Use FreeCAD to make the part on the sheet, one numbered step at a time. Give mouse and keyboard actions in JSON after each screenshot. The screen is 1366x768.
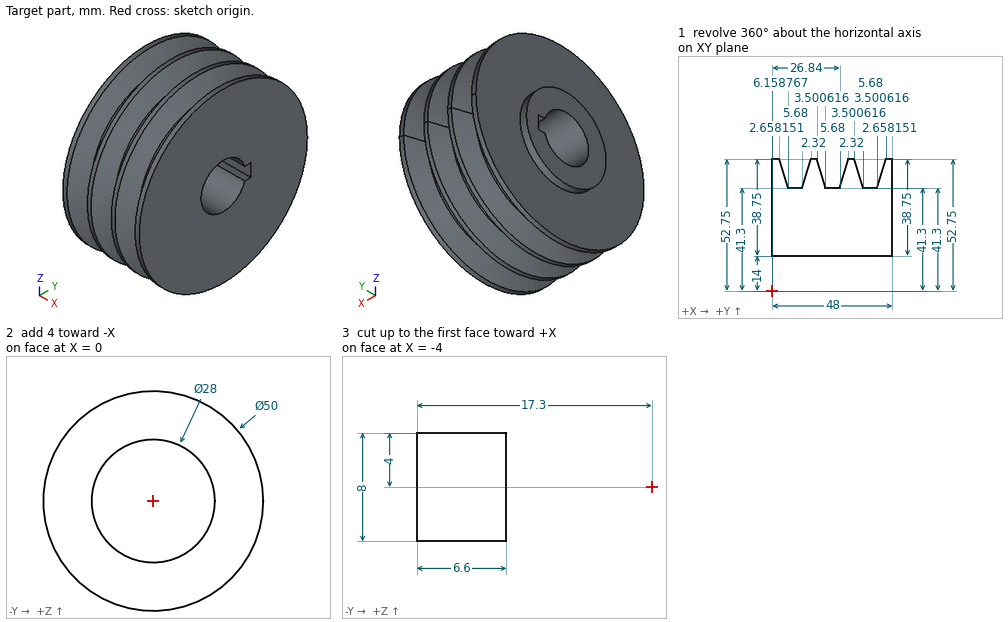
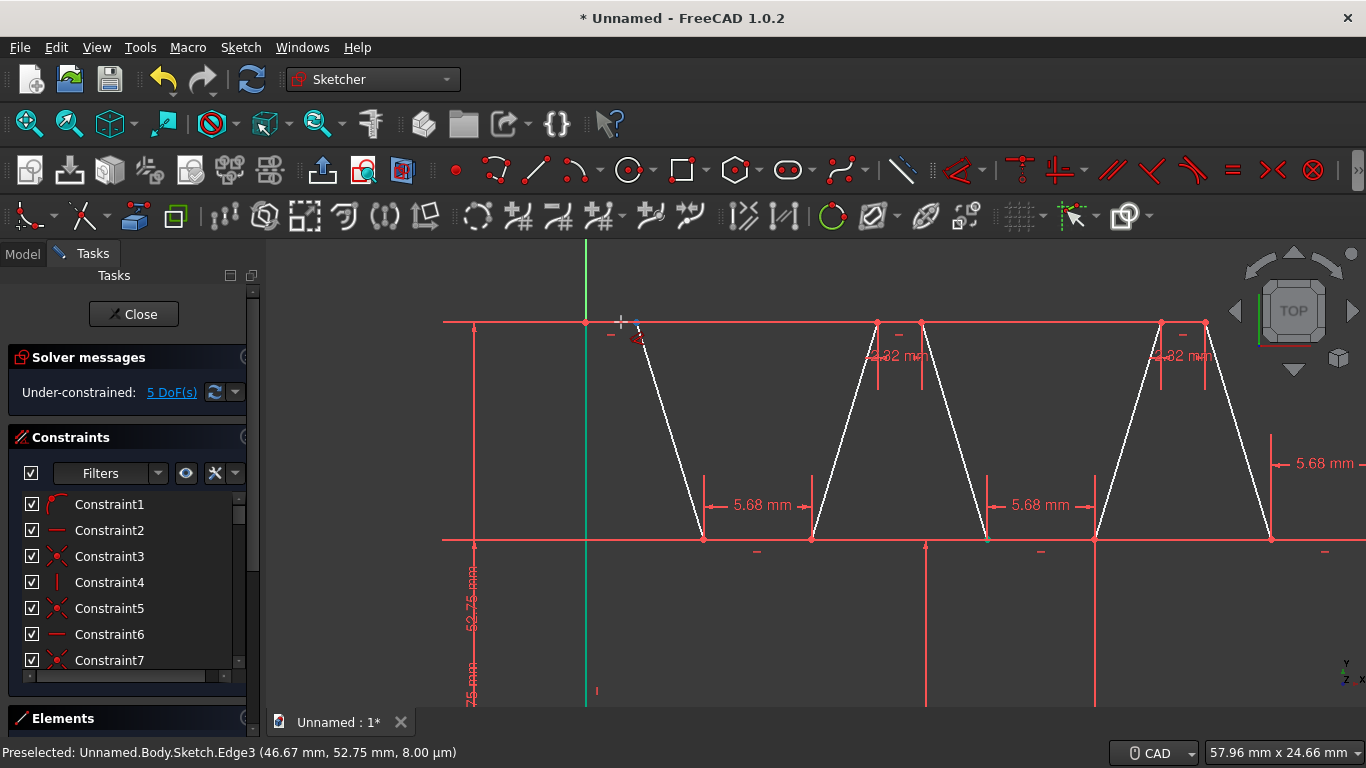
{"action": "left_click", "coordinate": [621, 322]}
{"action": "left_click", "coordinate": [611, 288]}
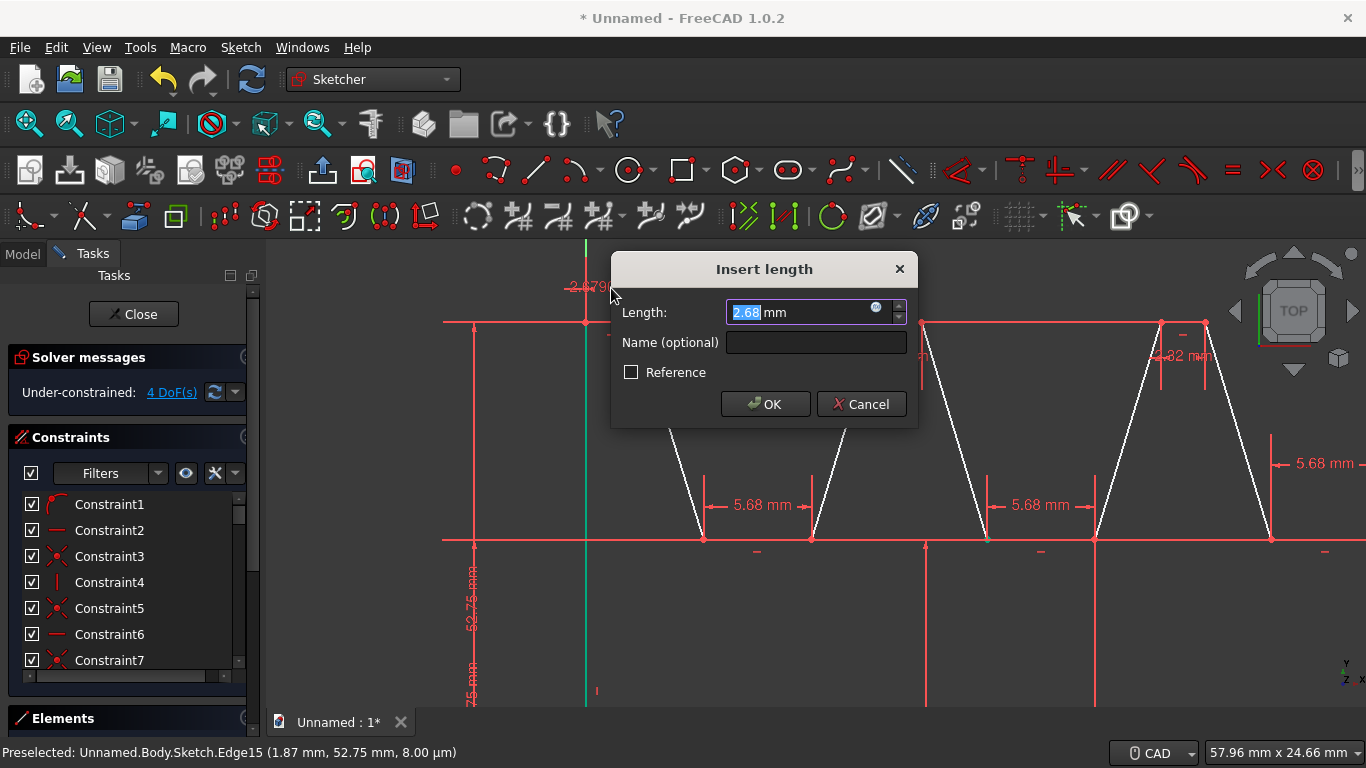
{"action": "type", "text": "2.658151"}
{"action": "key", "text": "Return"}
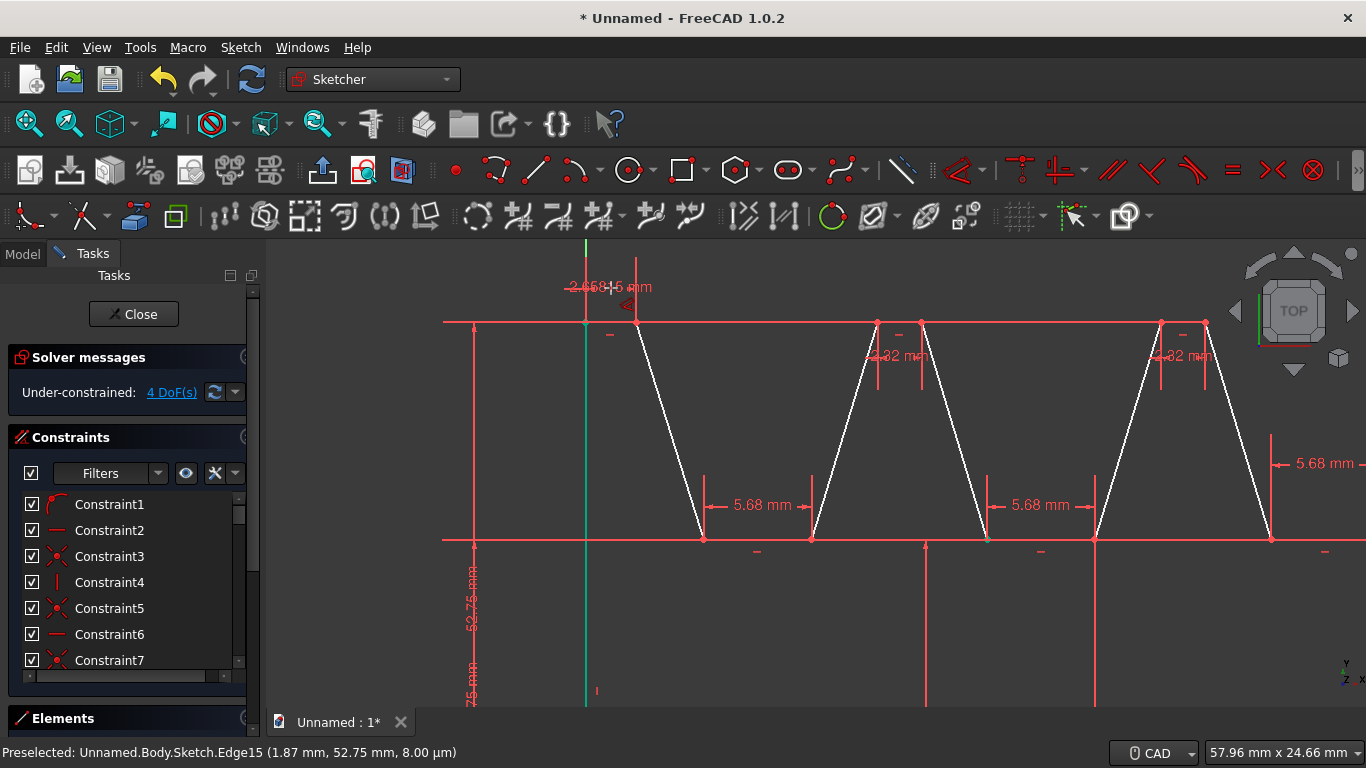
{"action": "left_click", "coordinate": [704, 540]}
{"action": "left_click", "coordinate": [645, 506]}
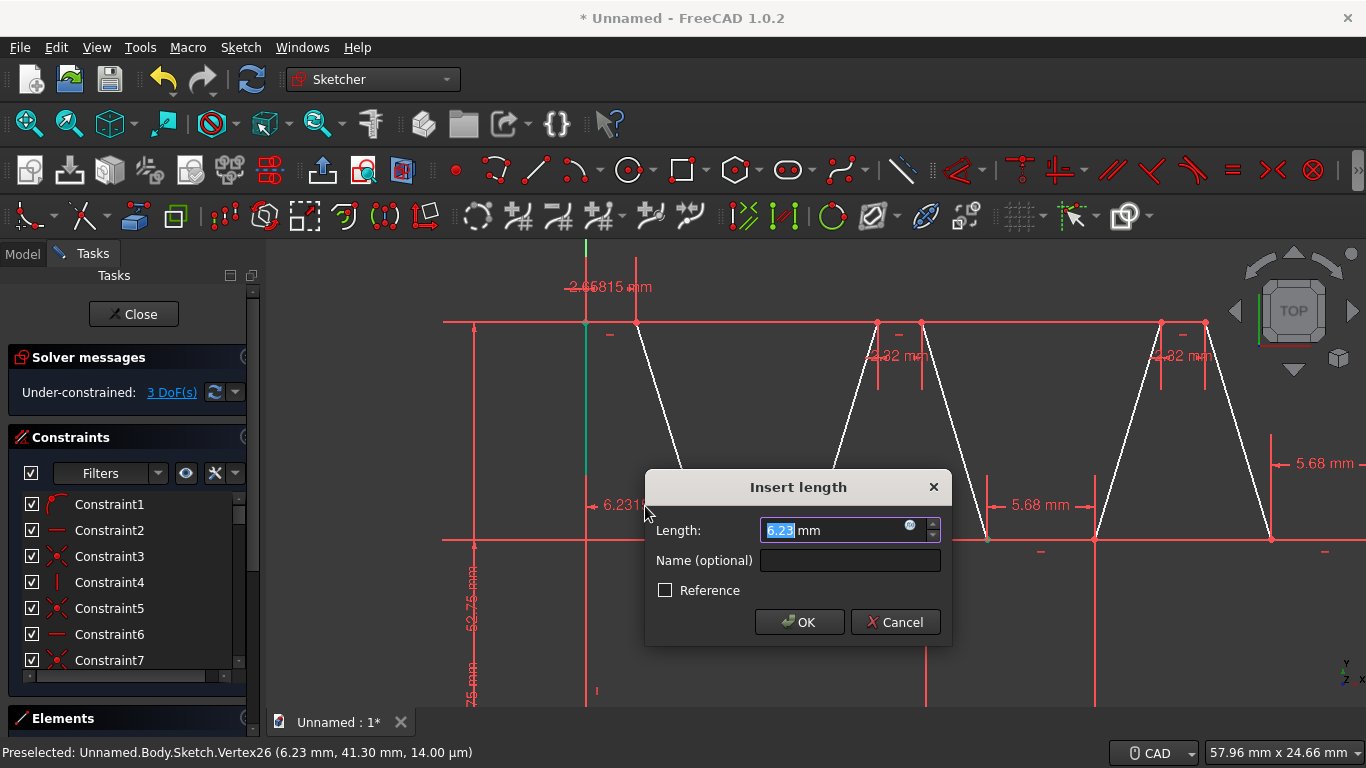
{"action": "type", "text": "6.158767"}
{"action": "key", "text": "Return"}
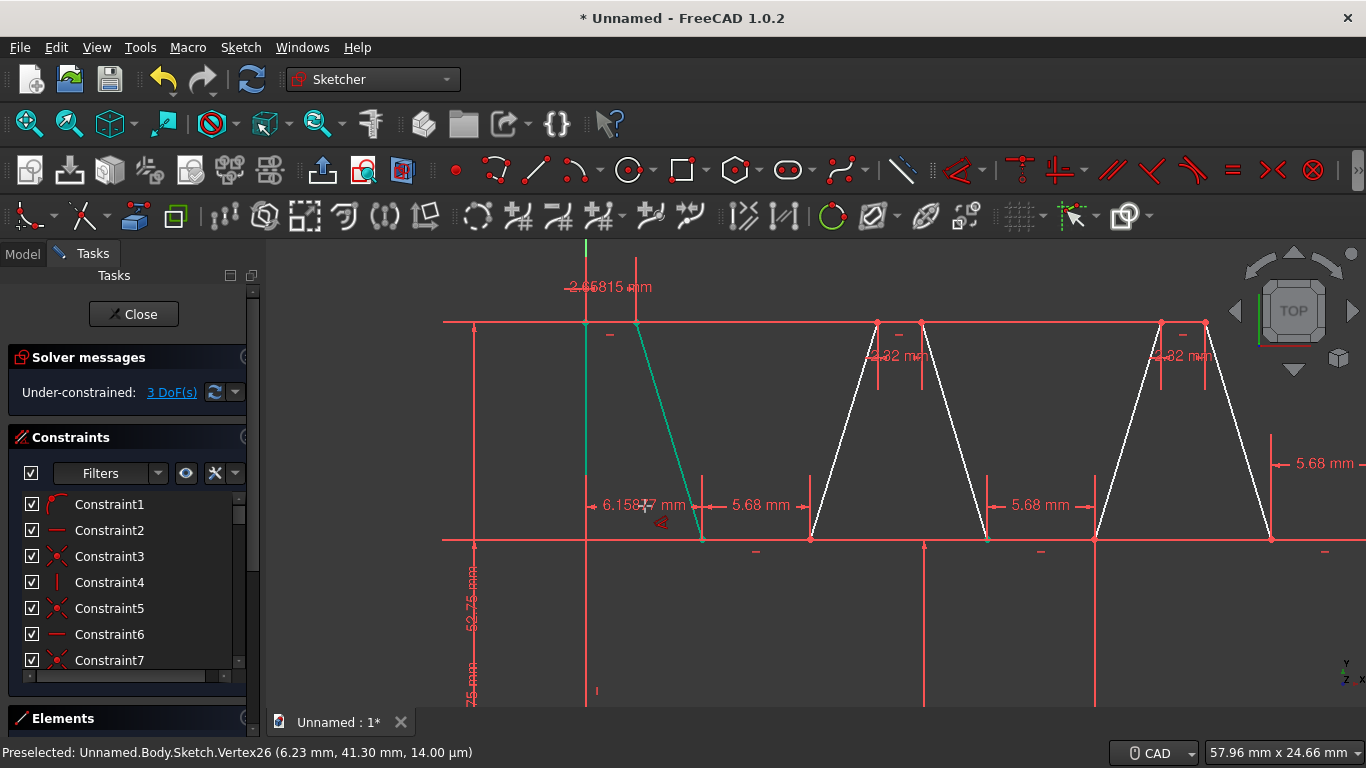
{"action": "scroll", "coordinate": [621, 322], "scroll_direction": "down", "scroll_amount": 6}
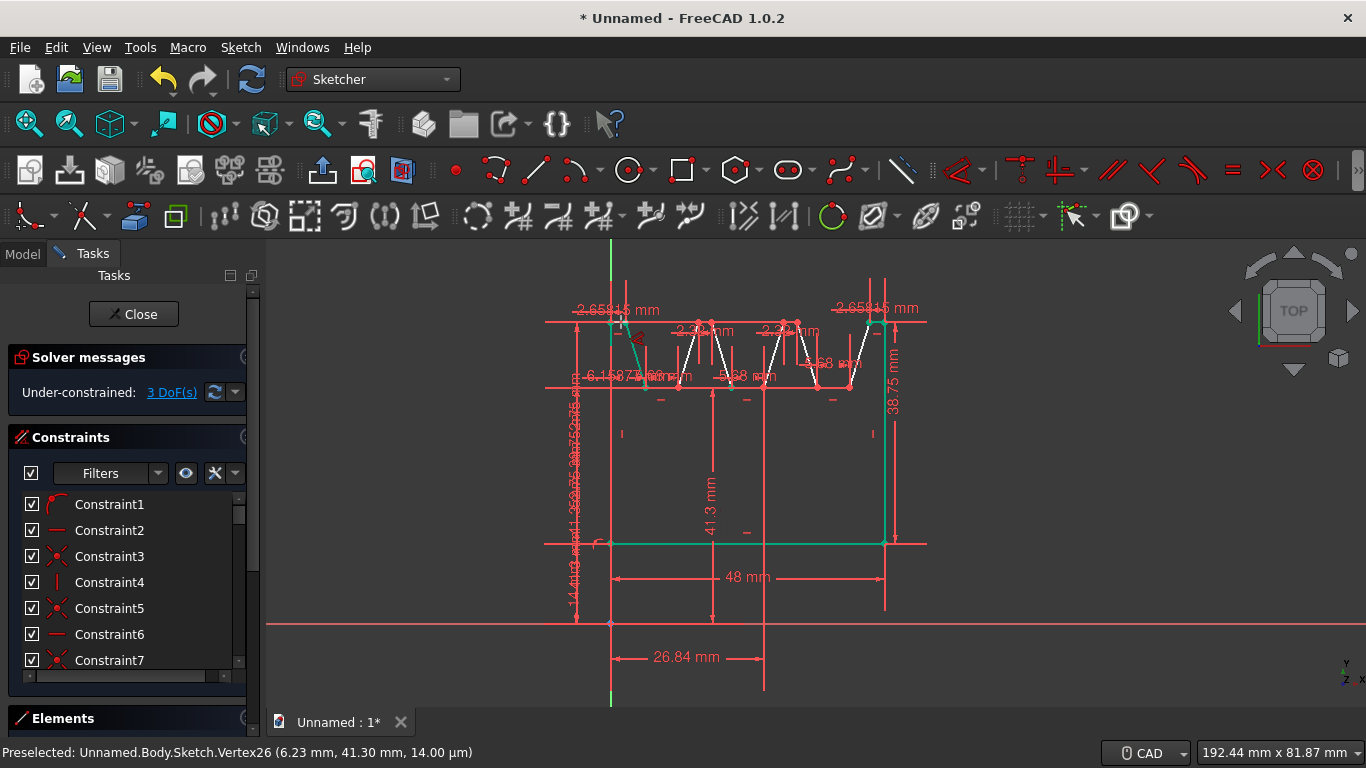
{"action": "scroll", "coordinate": [864, 342], "scroll_direction": "up", "scroll_amount": 4}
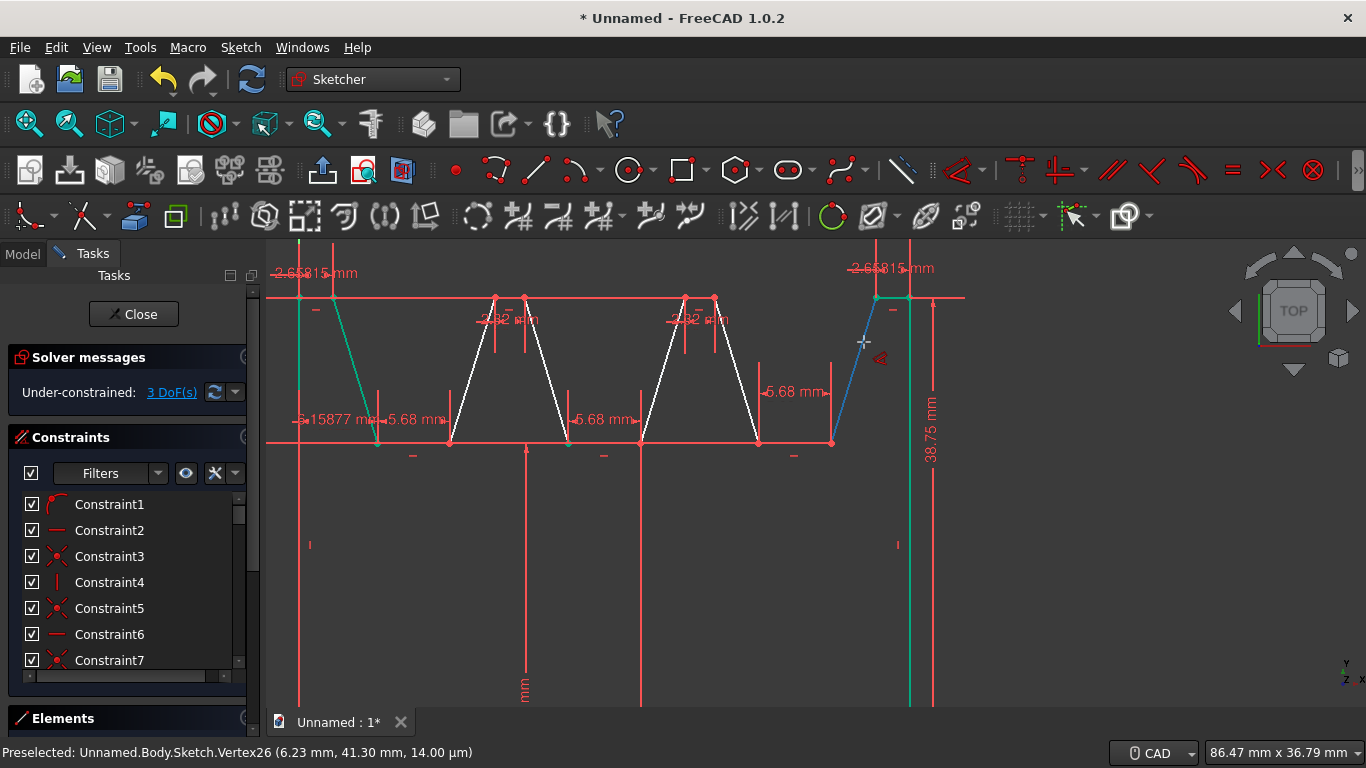
{"action": "left_click", "coordinate": [863, 342]}
{"action": "left_click", "coordinate": [854, 477]}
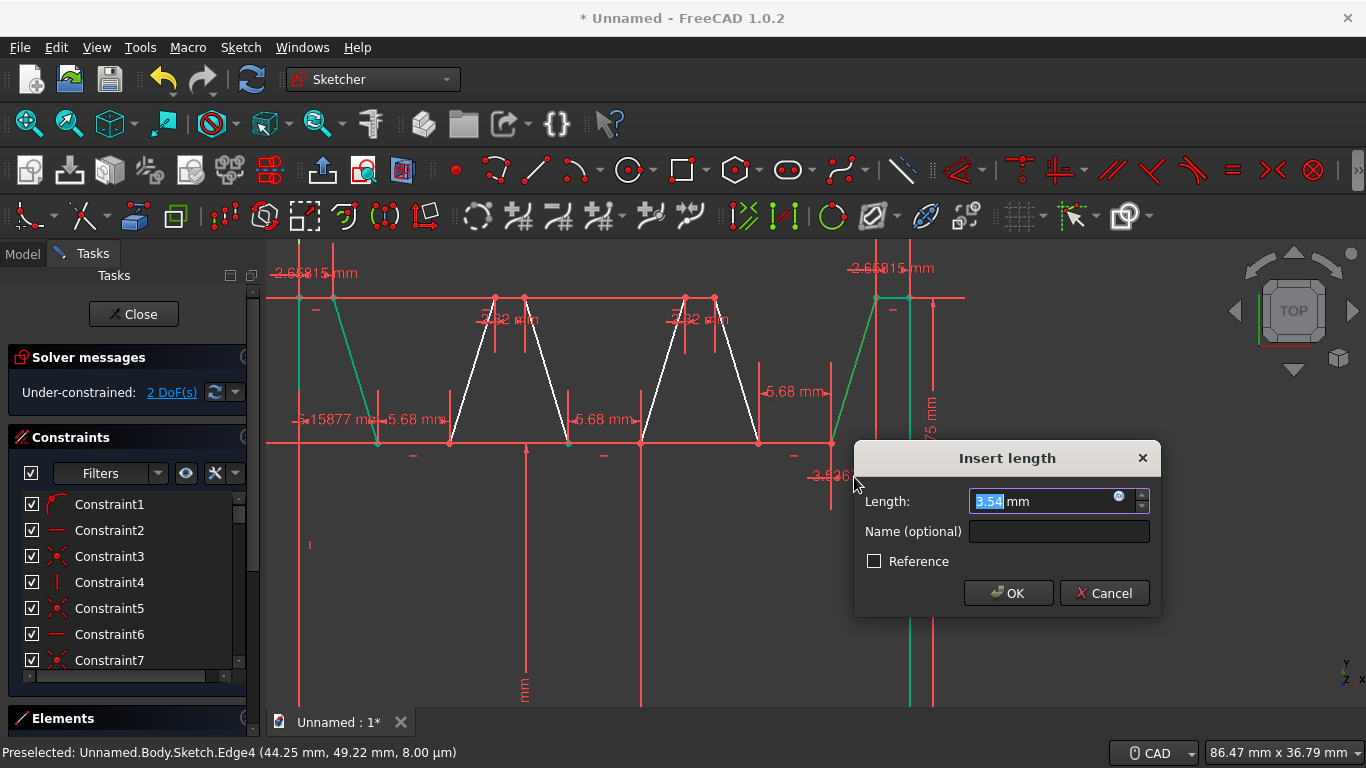
{"action": "type", "text": "3.500616"}
{"action": "key", "text": "Return"}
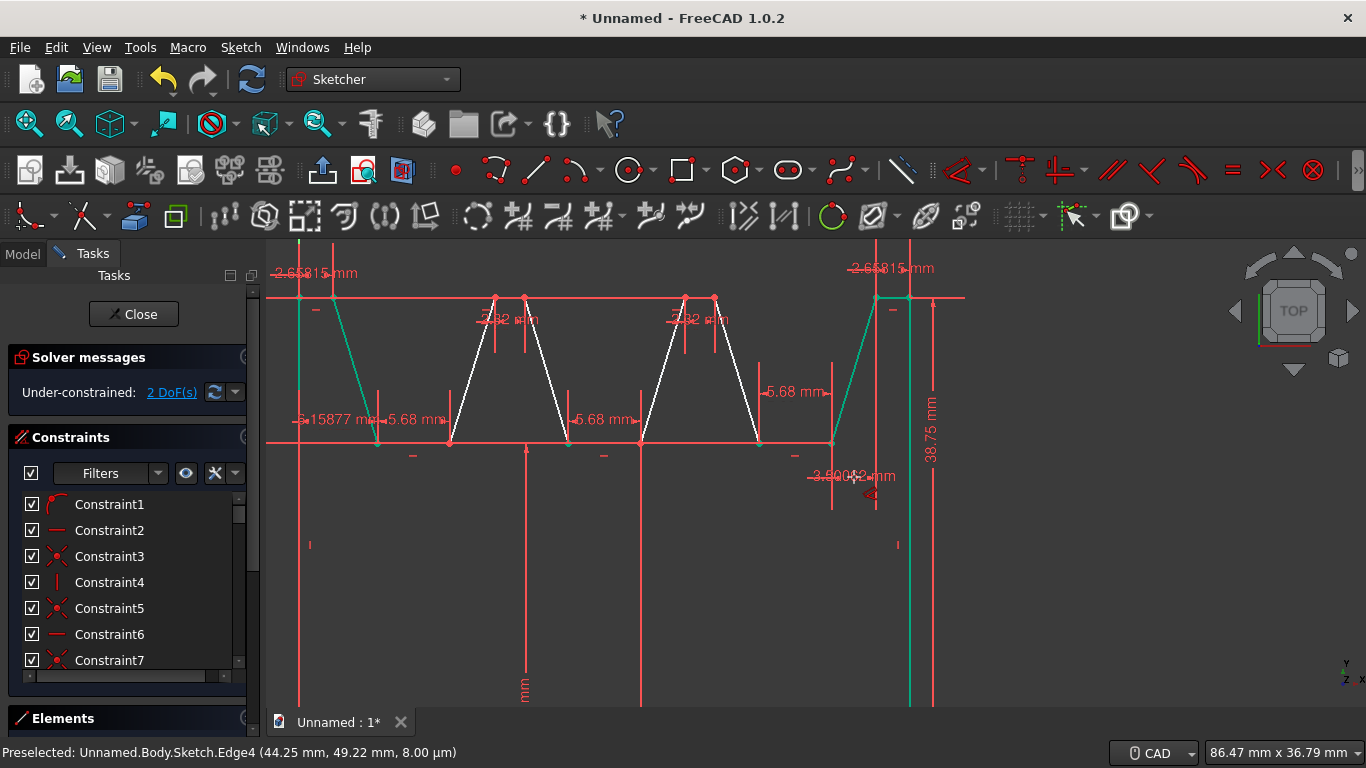
{"action": "left_click", "coordinate": [746, 400]}
{"action": "left_click", "coordinate": [737, 477]}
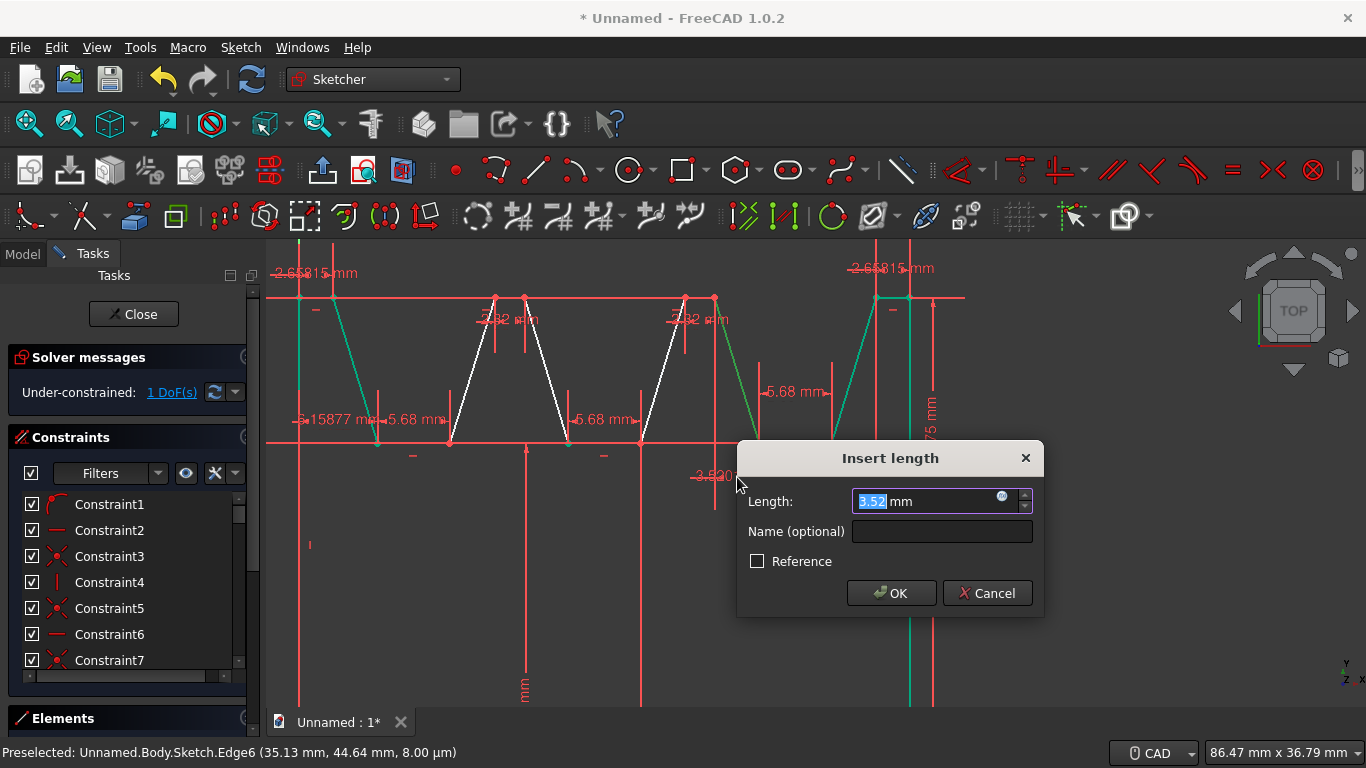
{"action": "type", "text": "3.500616"}
{"action": "key", "text": "Return"}